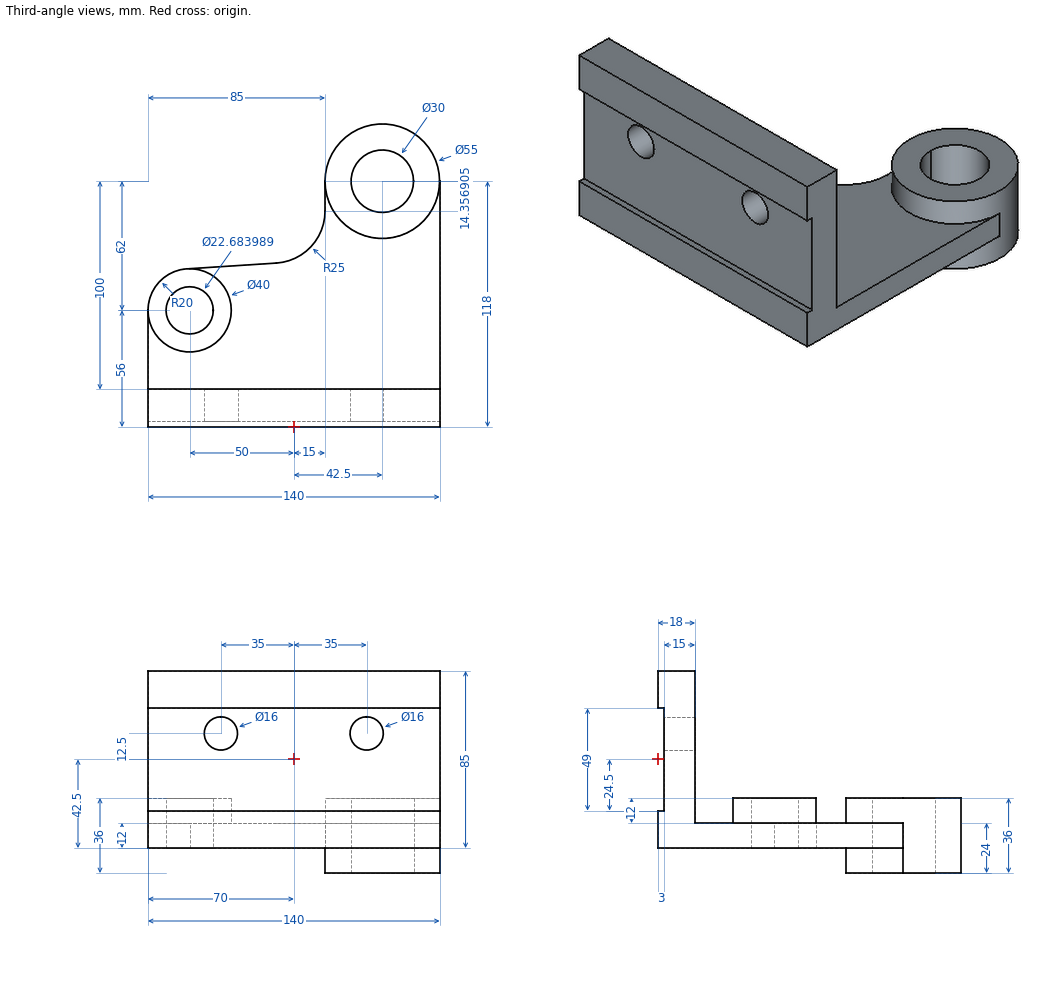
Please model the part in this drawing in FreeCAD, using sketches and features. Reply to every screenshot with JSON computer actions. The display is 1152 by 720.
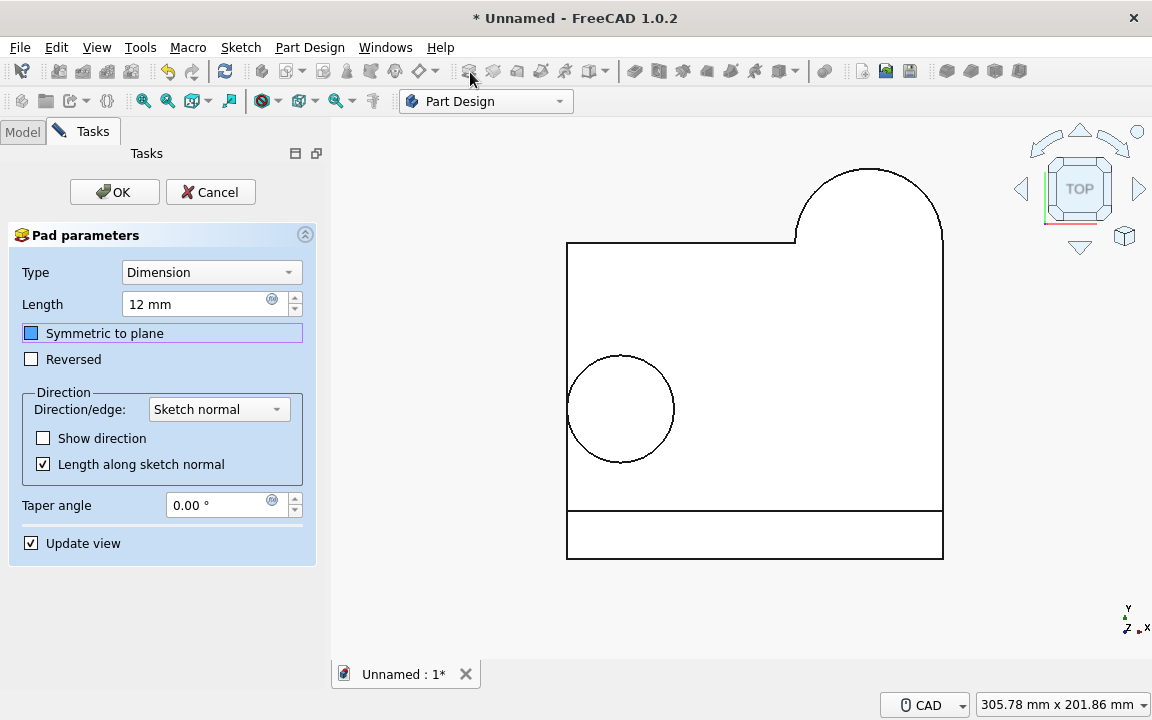
{"action": "left_click", "coordinate": [30, 359]}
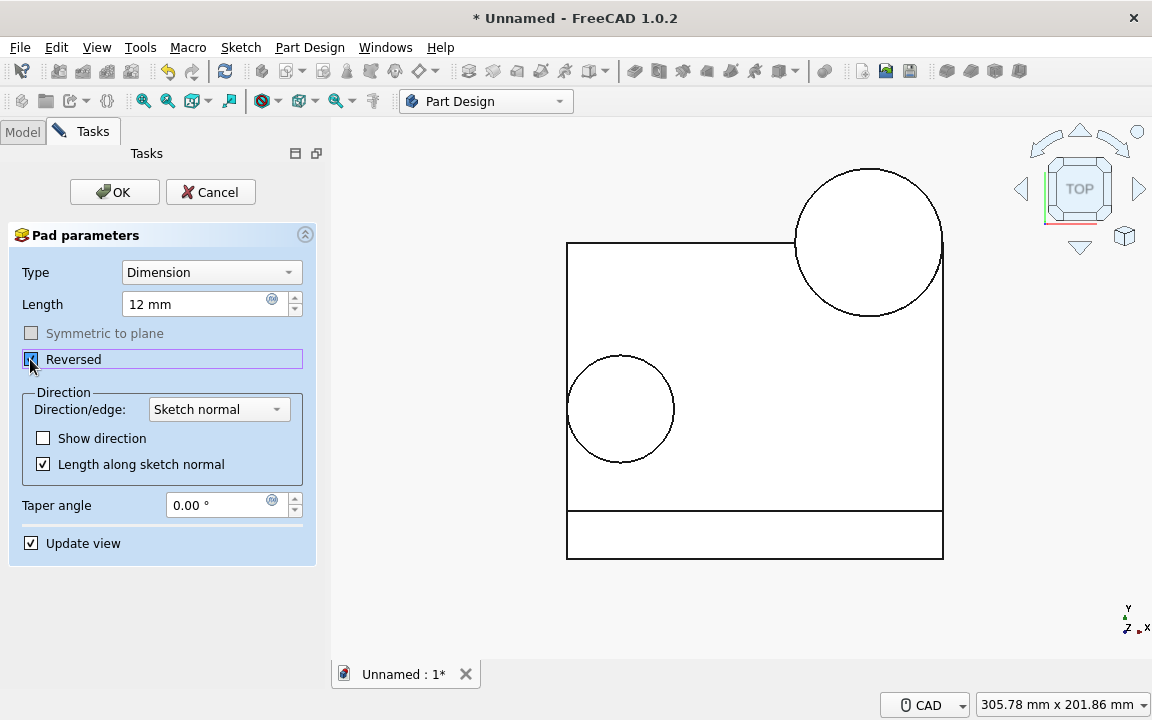
{"action": "left_click", "coordinate": [115, 192]}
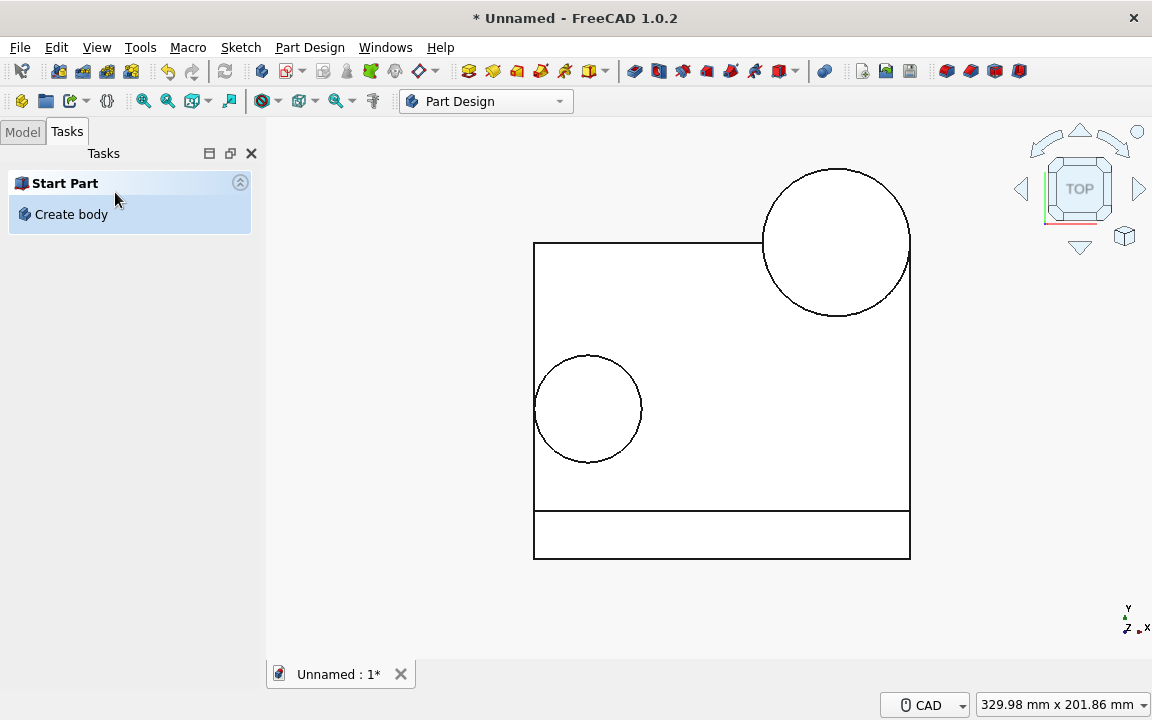
{"action": "key", "text": "5"}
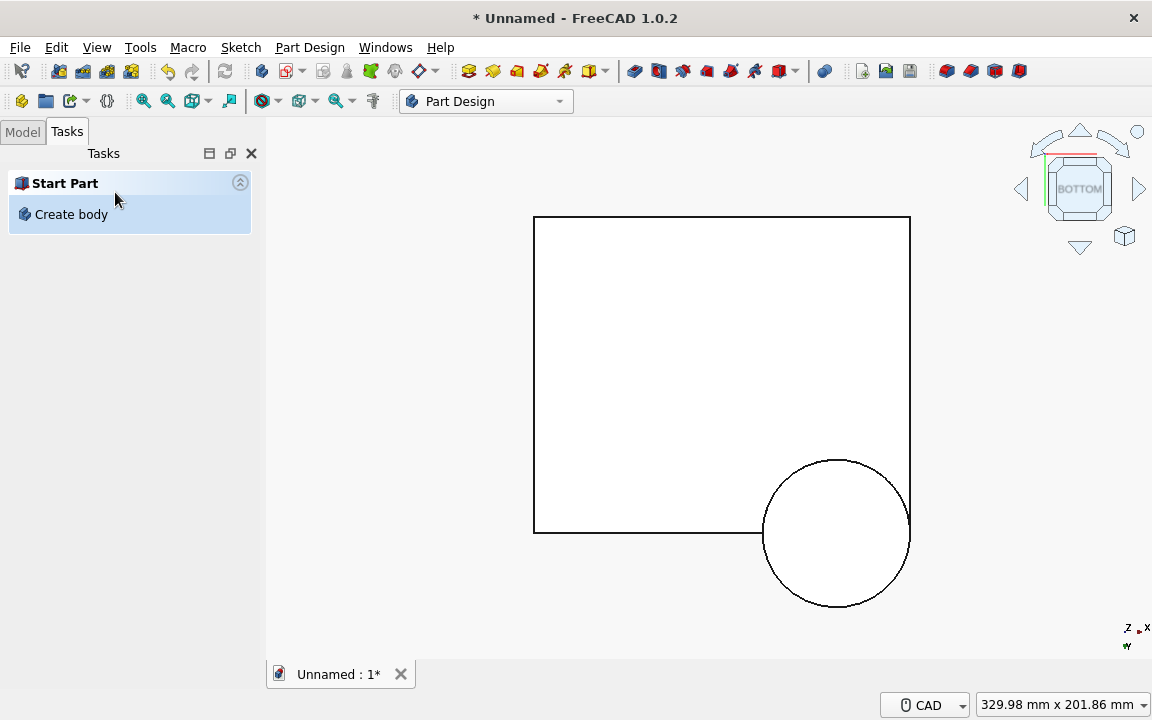
{"action": "left_click", "coordinate": [669, 374]}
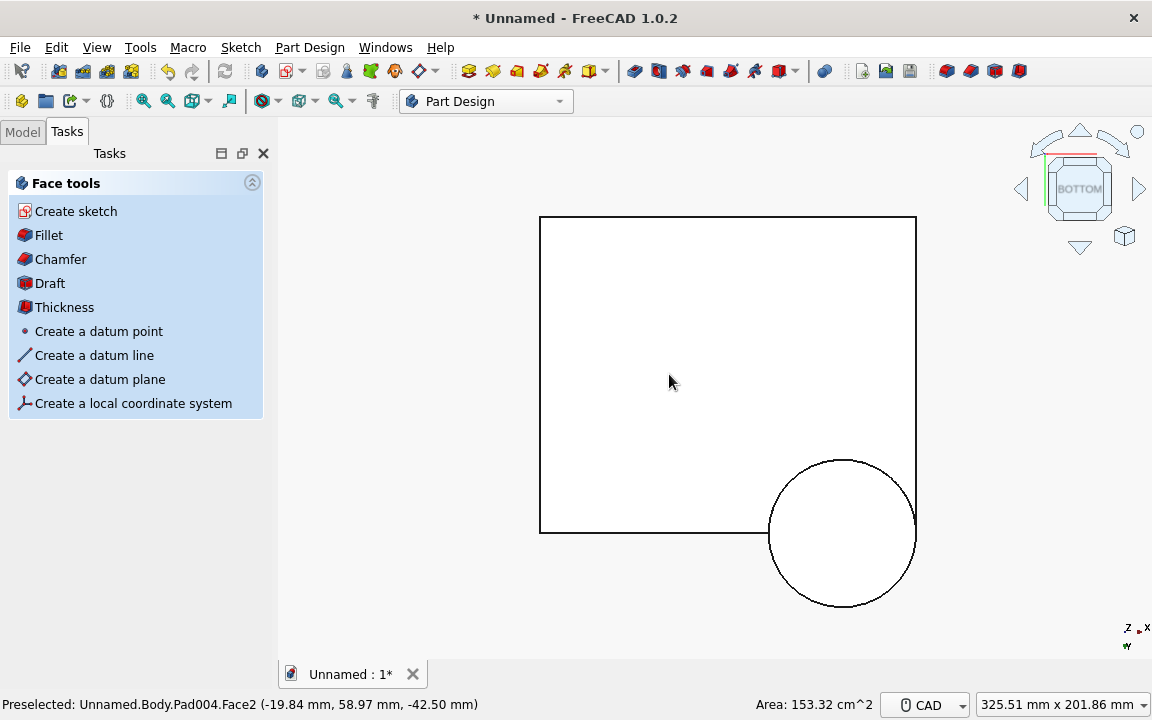
{"action": "left_click", "coordinate": [286, 72]}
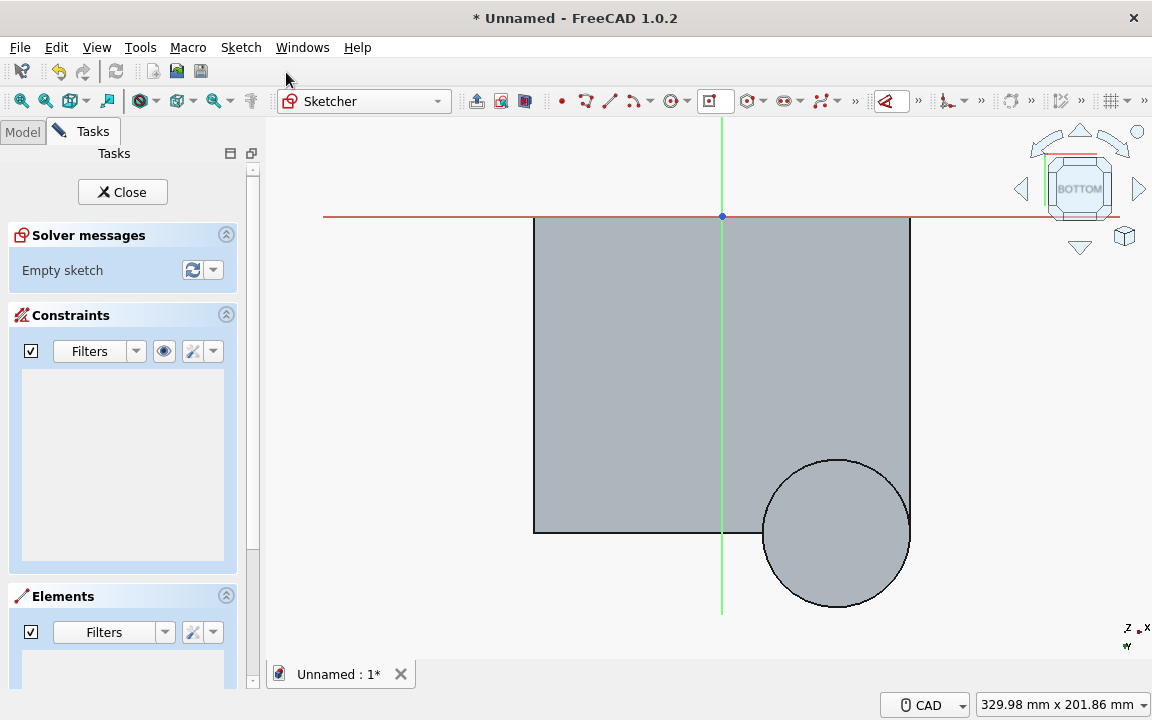
{"action": "key", "text": "q s"}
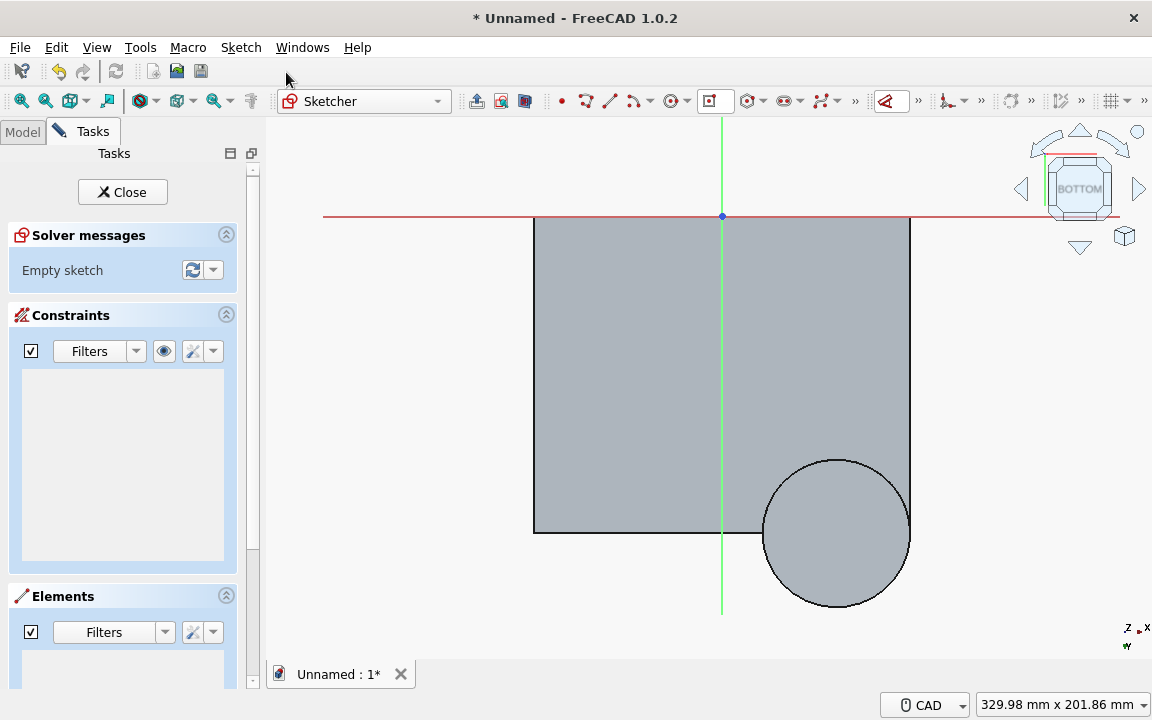
{"action": "left_click", "coordinate": [586, 102]}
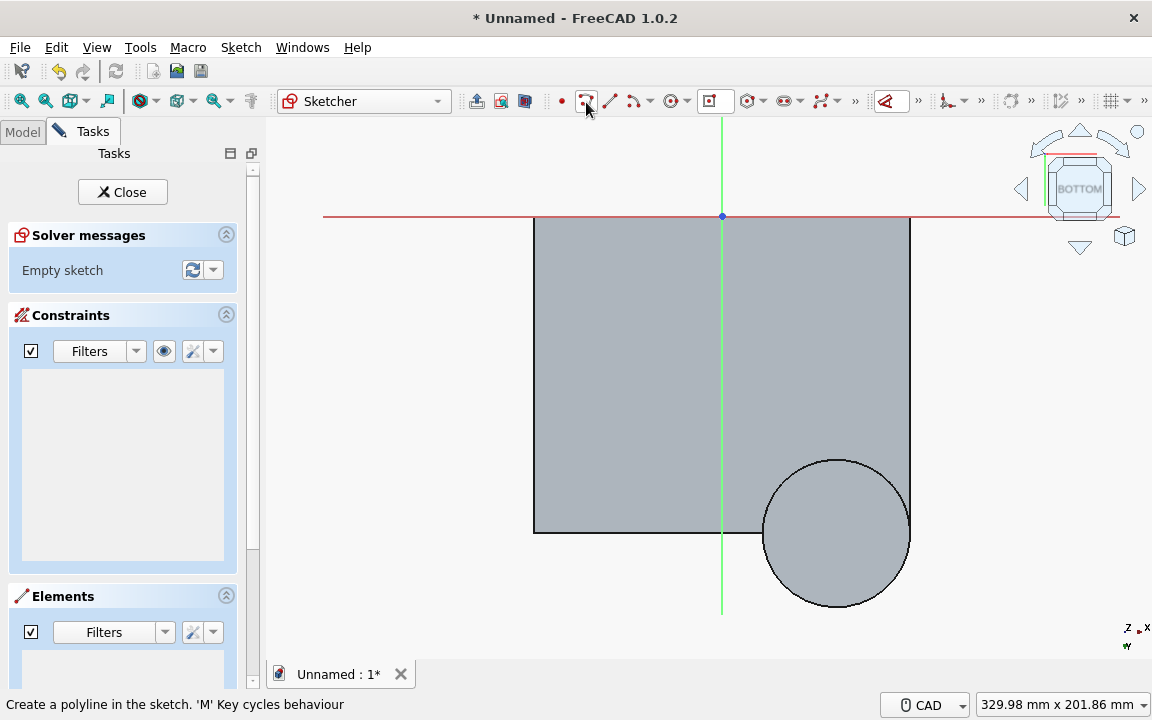
{"action": "left_click", "coordinate": [763, 495]}
{"action": "left_click", "coordinate": [763, 533]}
{"action": "left_click", "coordinate": [534, 533]}
{"action": "left_click", "coordinate": [534, 367]}
{"action": "right_click", "coordinate": [534, 367]}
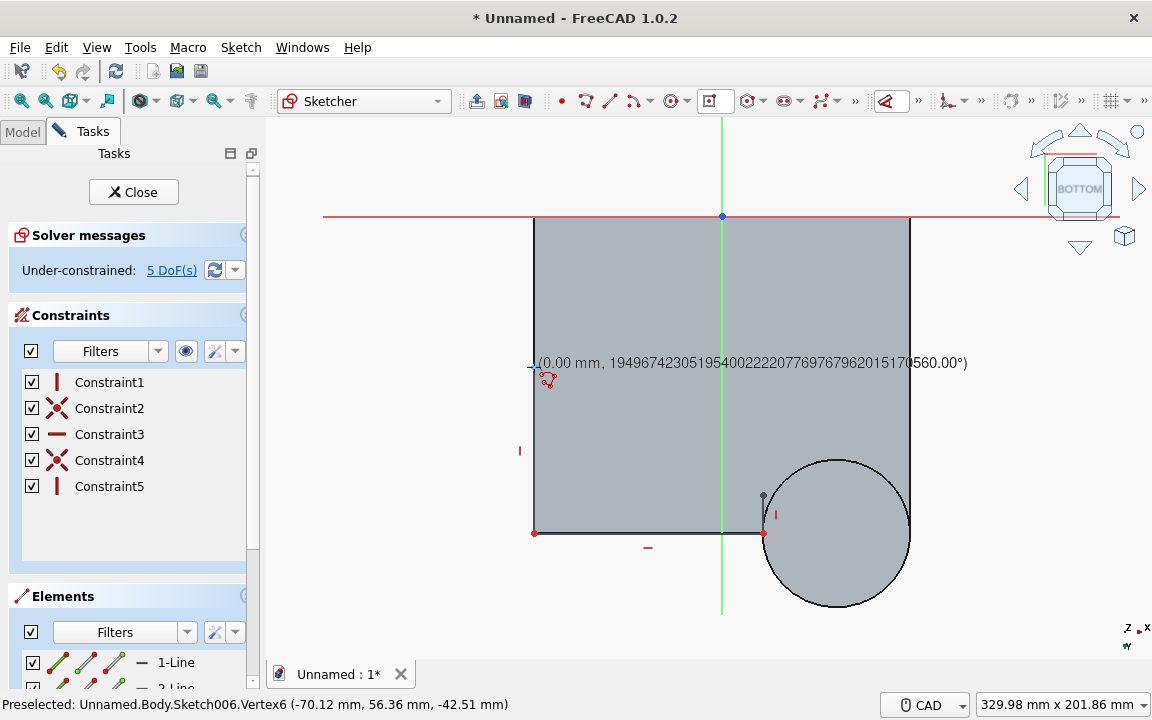
{"action": "left_click", "coordinate": [610, 102]}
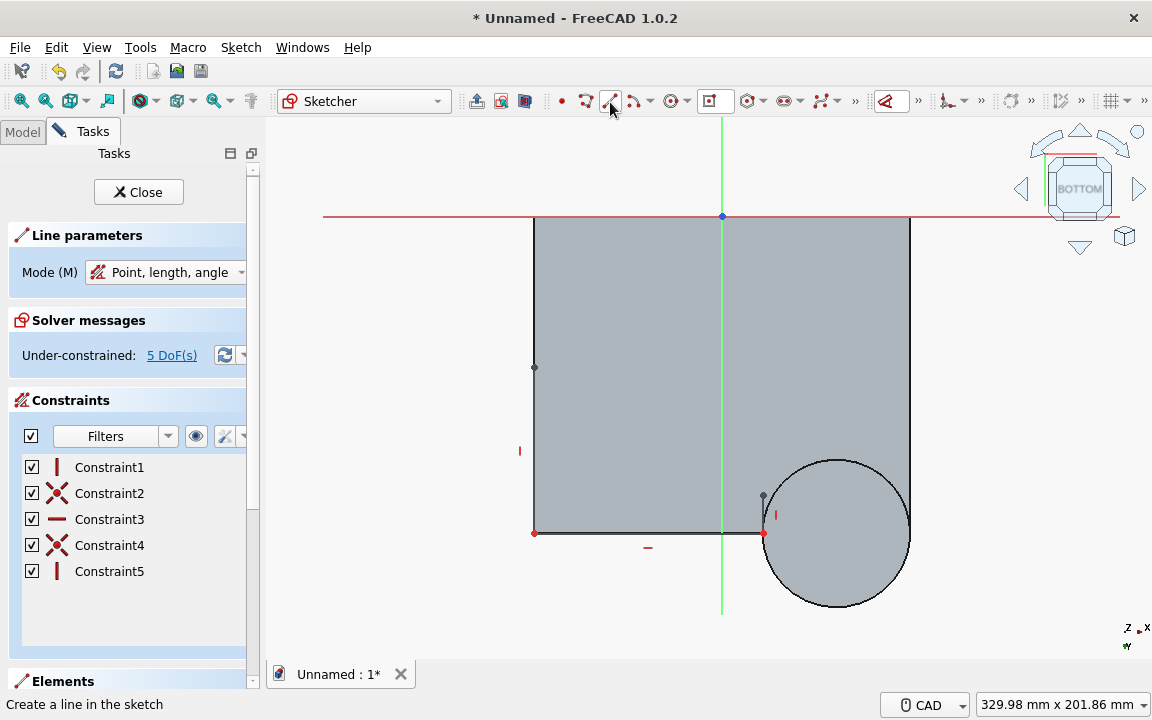
{"action": "left_click", "coordinate": [588, 421]}
{"action": "left_click", "coordinate": [700, 428]}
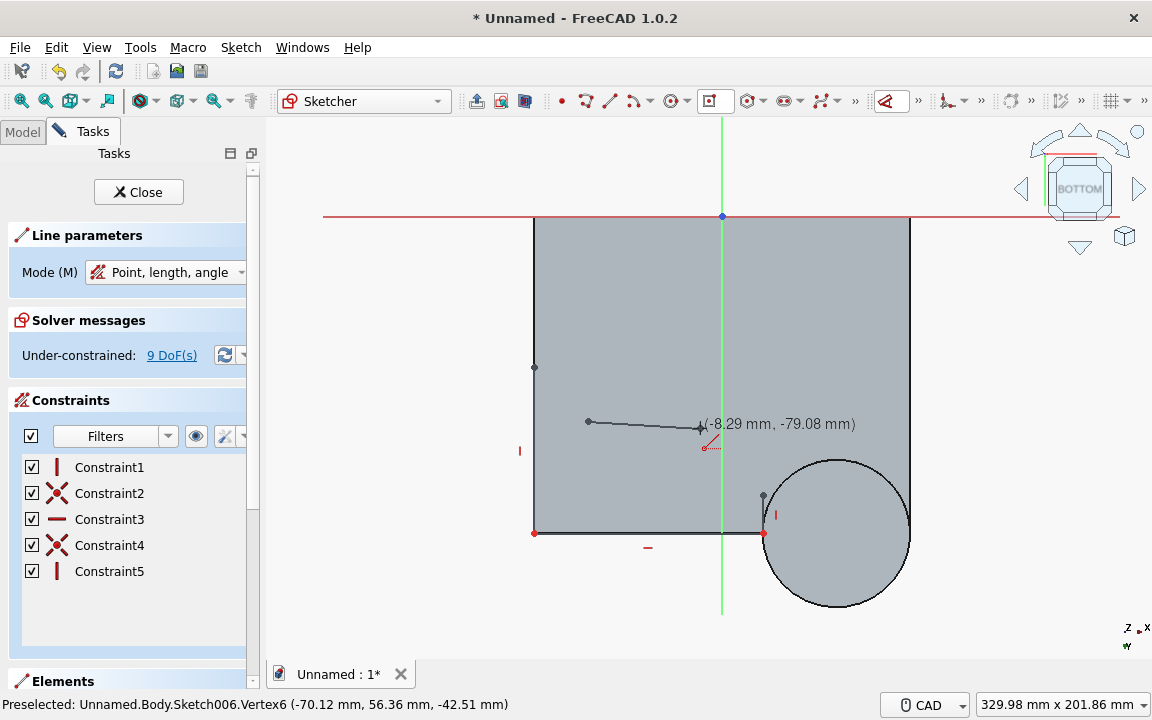
{"action": "key", "text": "g 3 a"}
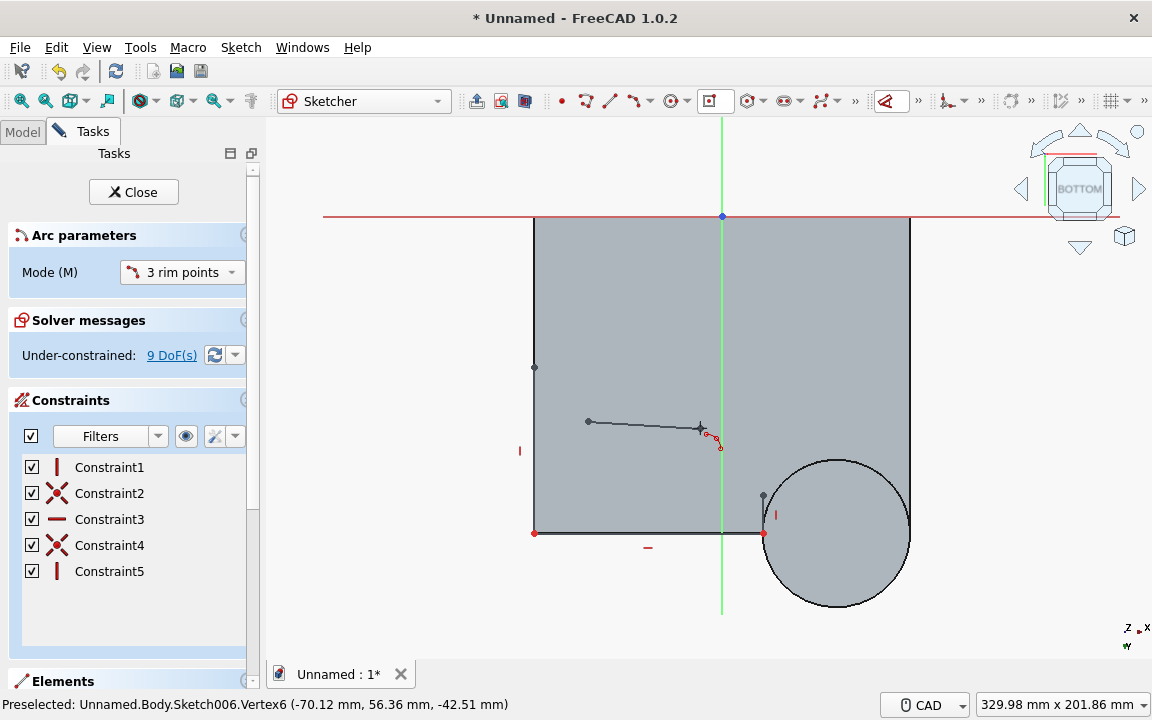
{"action": "left_click", "coordinate": [534, 368]}
{"action": "left_click", "coordinate": [588, 422]}
{"action": "left_click", "coordinate": [550, 405]}